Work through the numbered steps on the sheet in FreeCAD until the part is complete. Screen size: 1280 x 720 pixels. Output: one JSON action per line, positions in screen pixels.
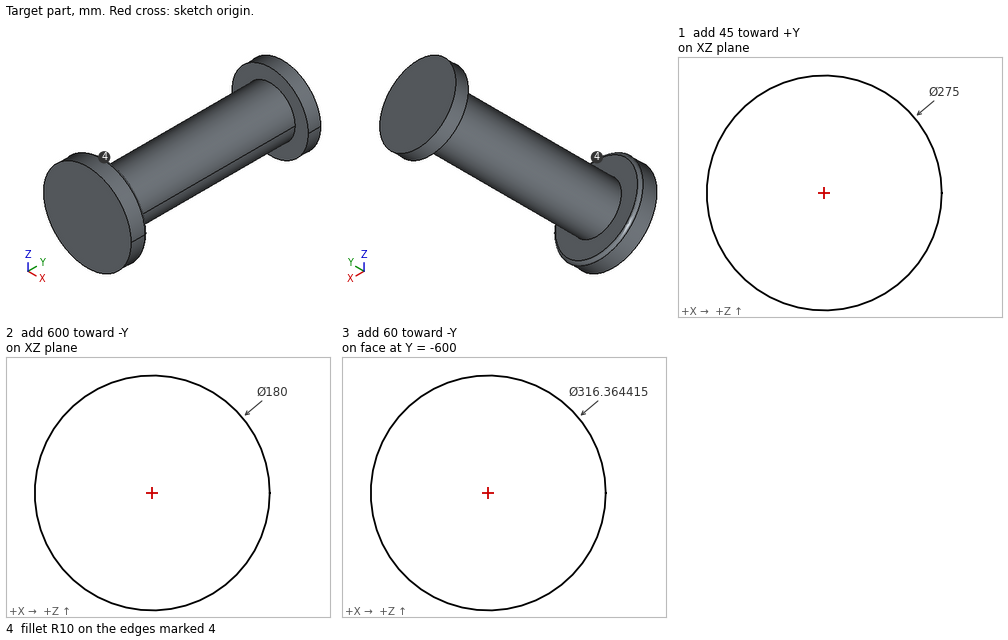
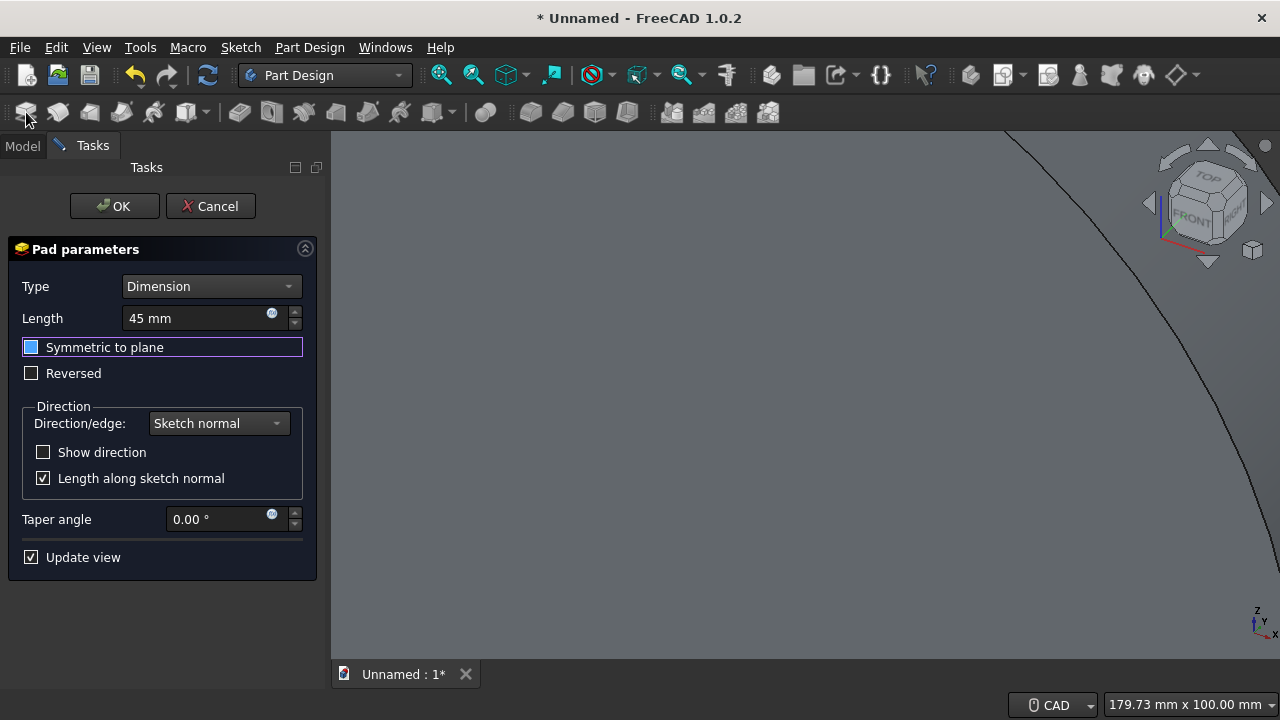
{"action": "left_click", "coordinate": [30, 373]}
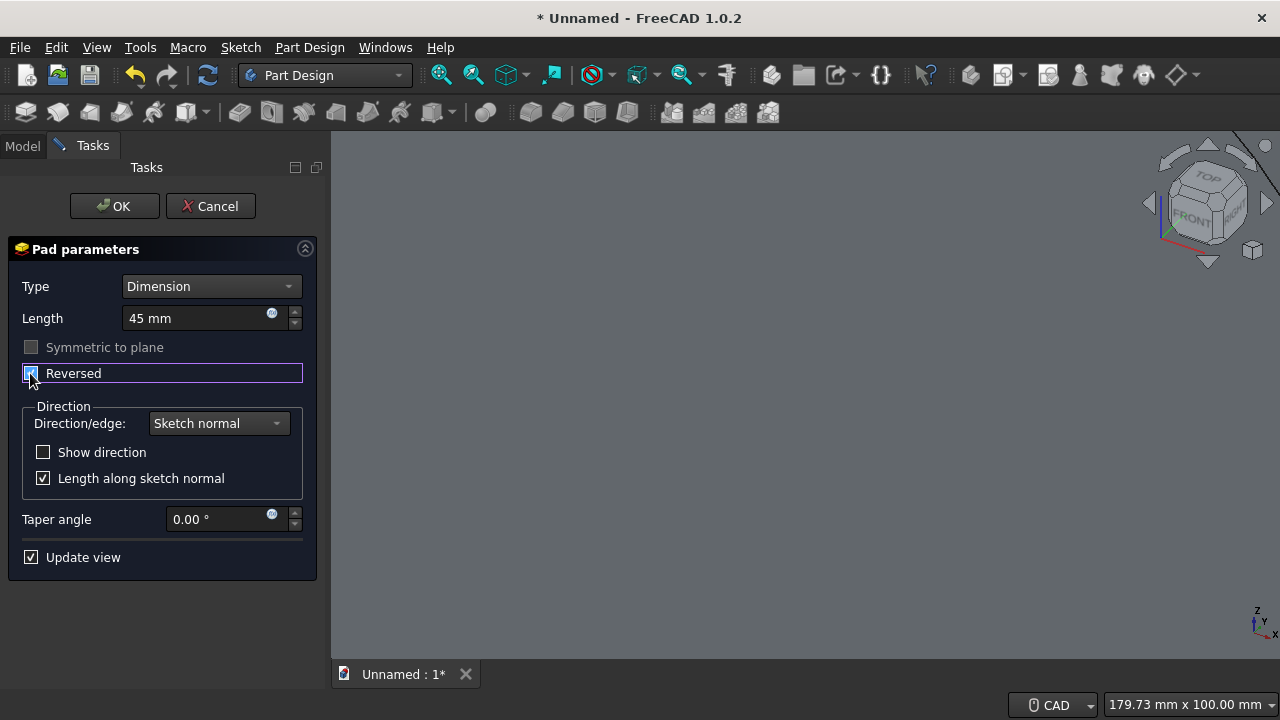
{"action": "left_click", "coordinate": [115, 206]}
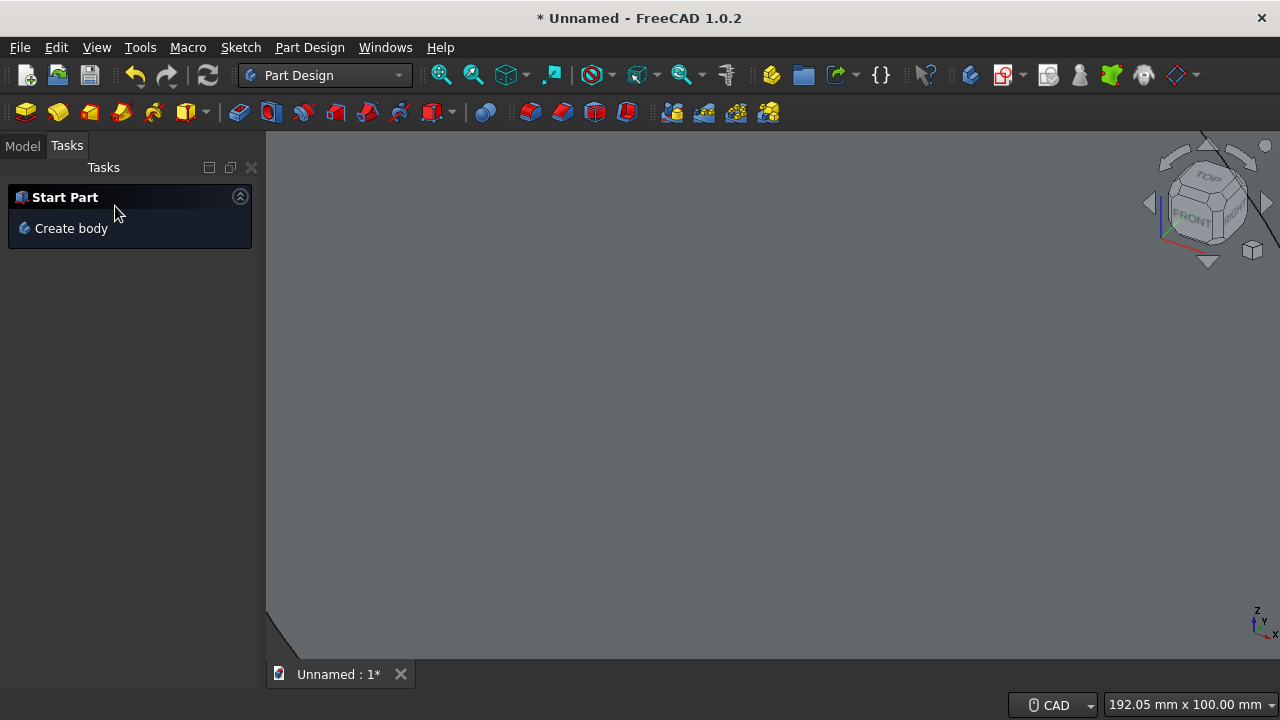
{"action": "key", "text": "v f"}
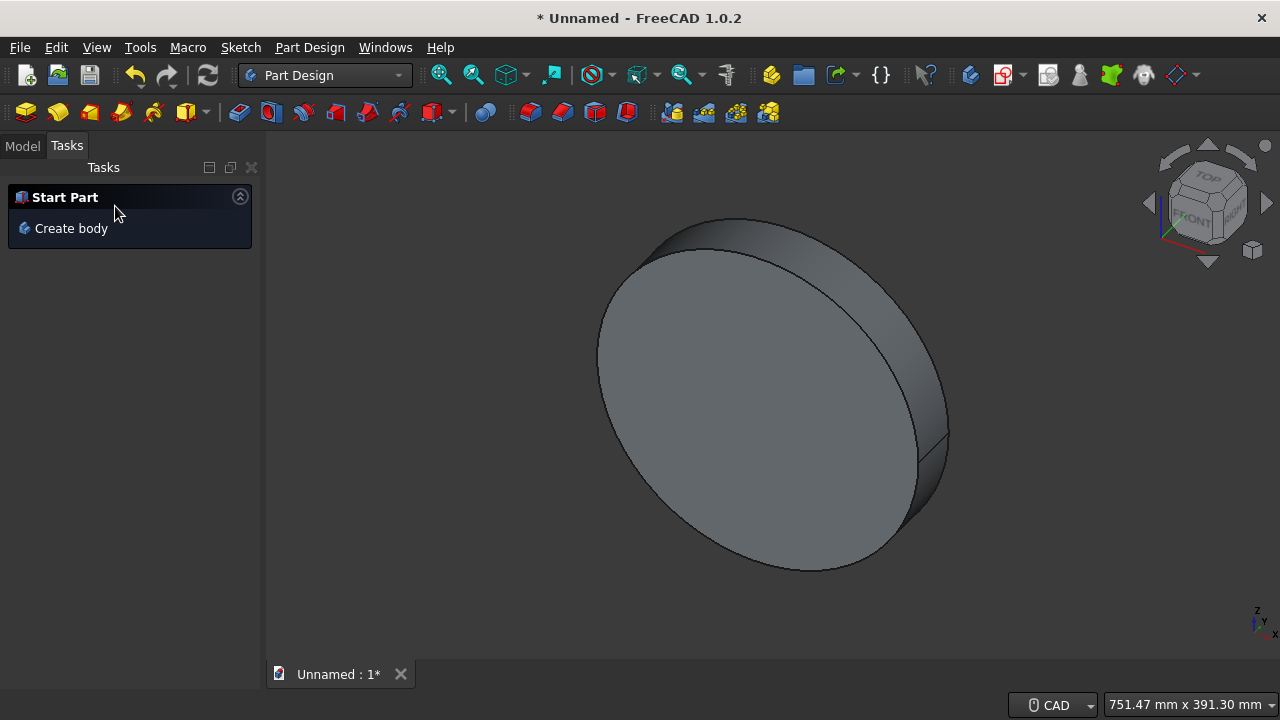
{"action": "left_click", "coordinate": [1004, 76]}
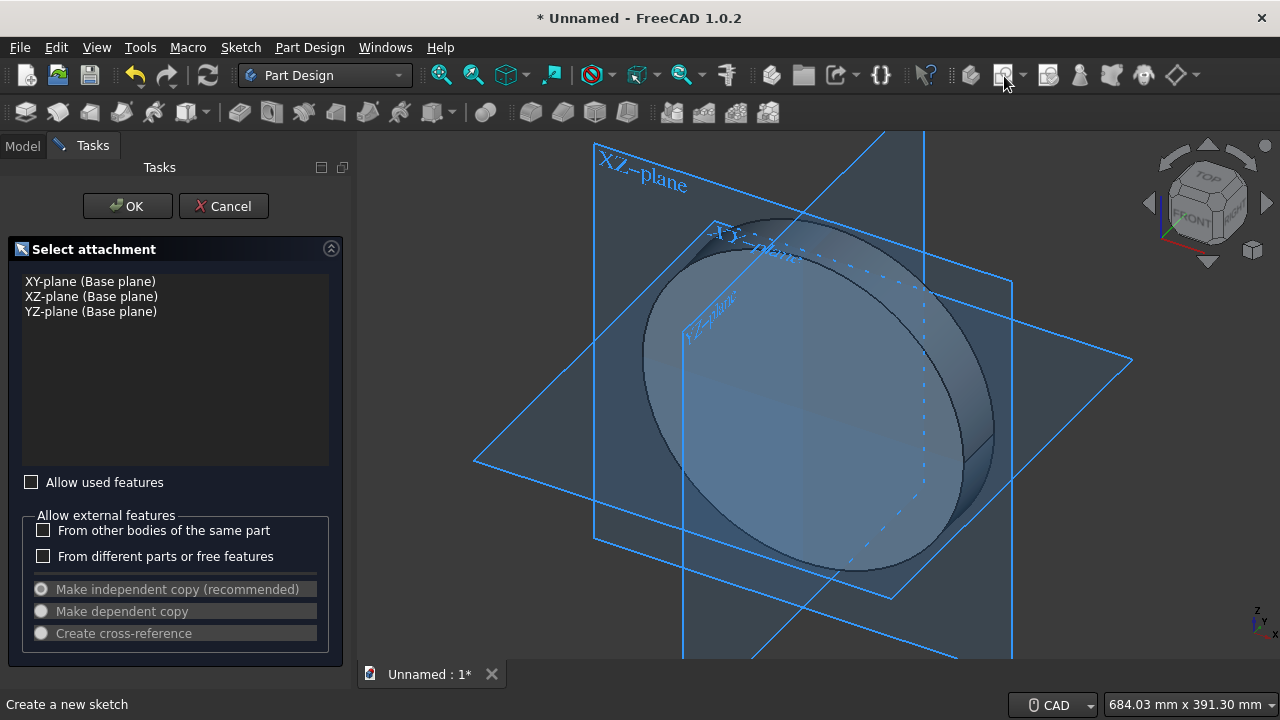
{"action": "left_click", "coordinate": [82, 296]}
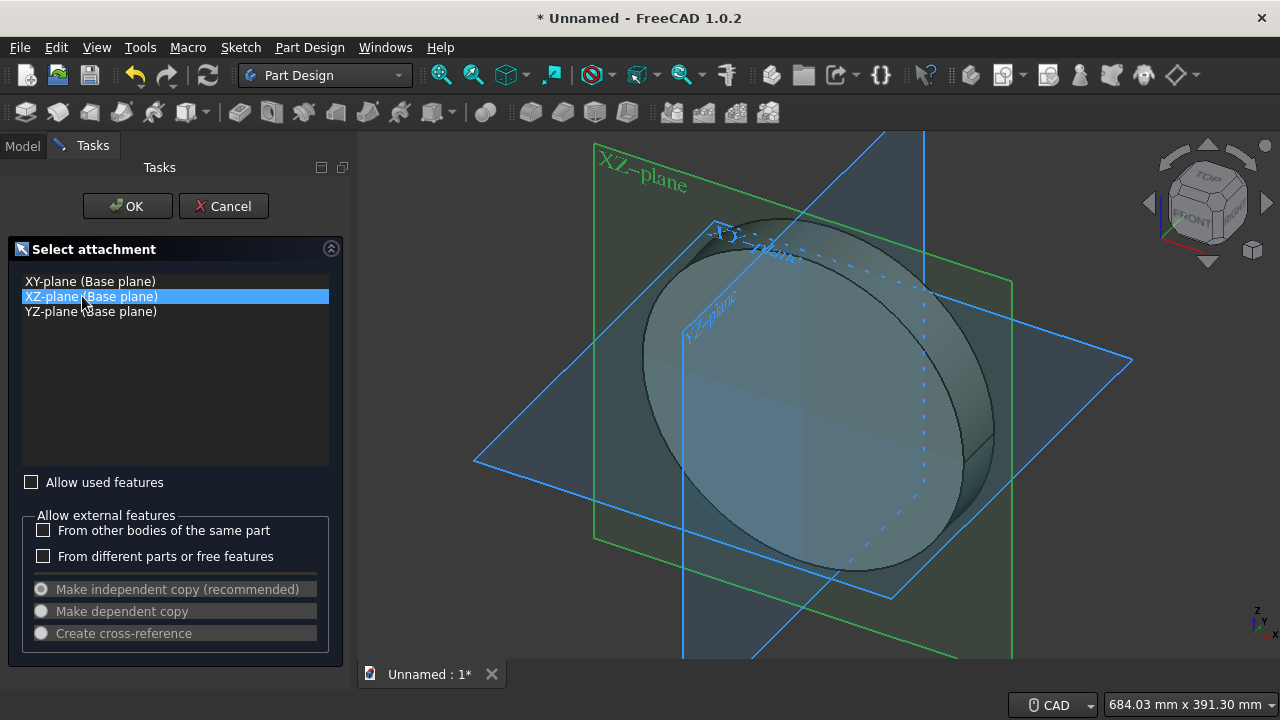
{"action": "left_click", "coordinate": [128, 206]}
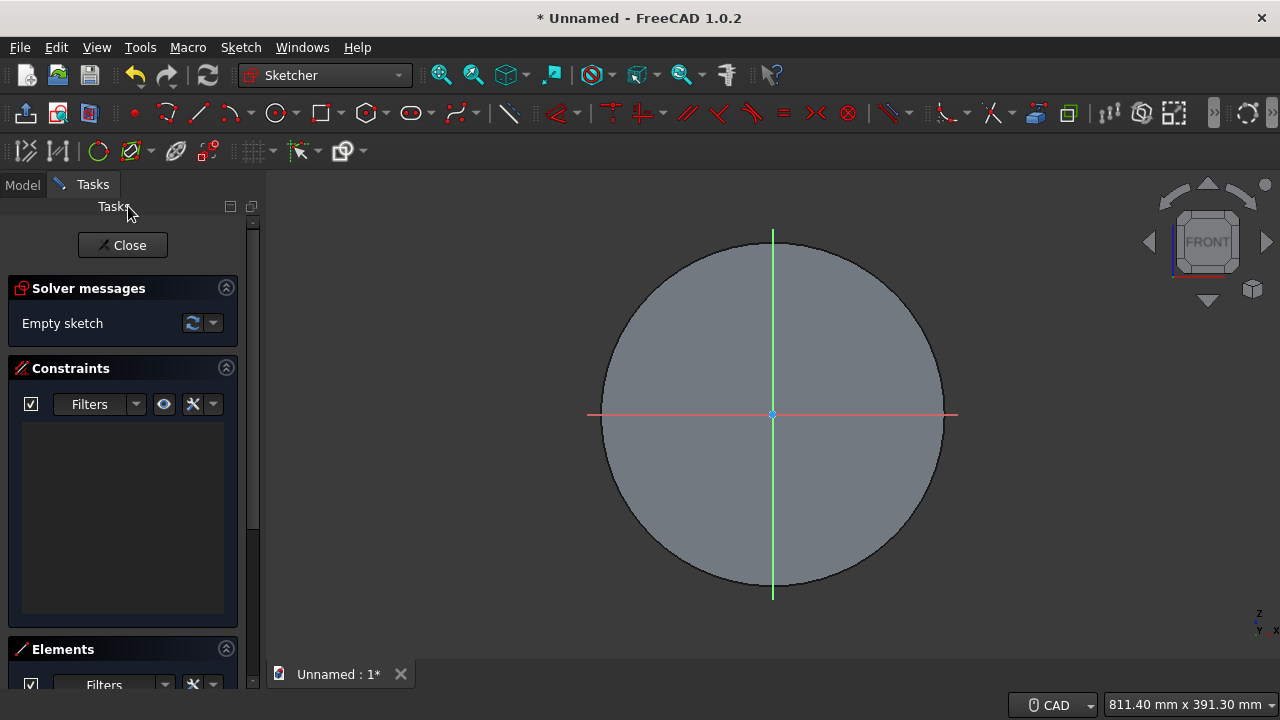
{"action": "scroll", "coordinate": [912, 414], "scroll_direction": "up", "scroll_amount": 2}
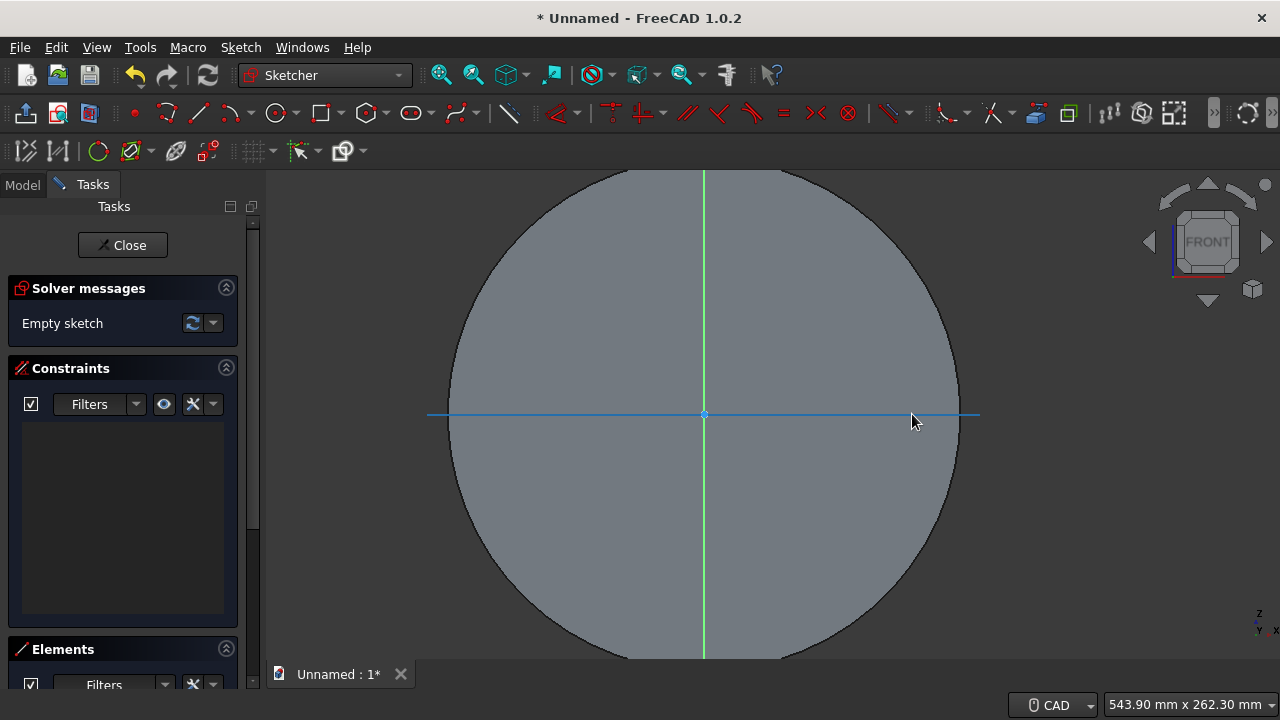
{"action": "key", "text": "g c"}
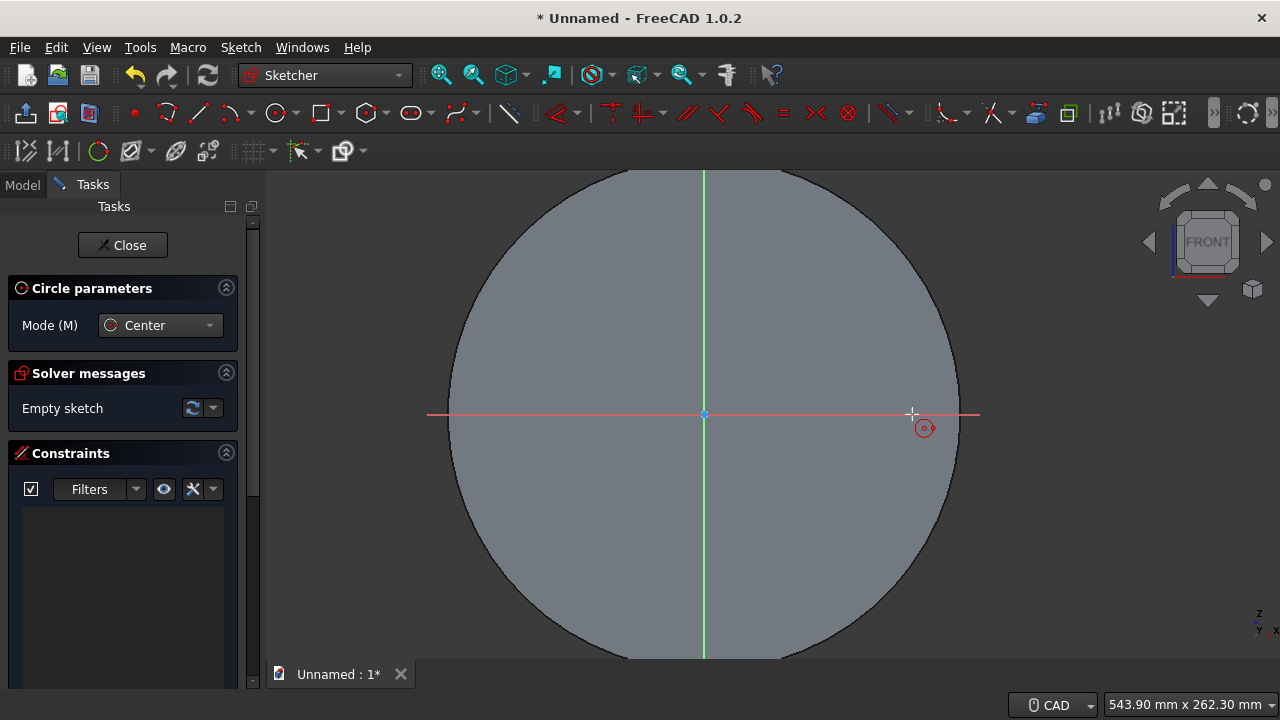
{"action": "left_click", "coordinate": [704, 414]}
{"action": "mouse_move", "coordinate": [823, 296]}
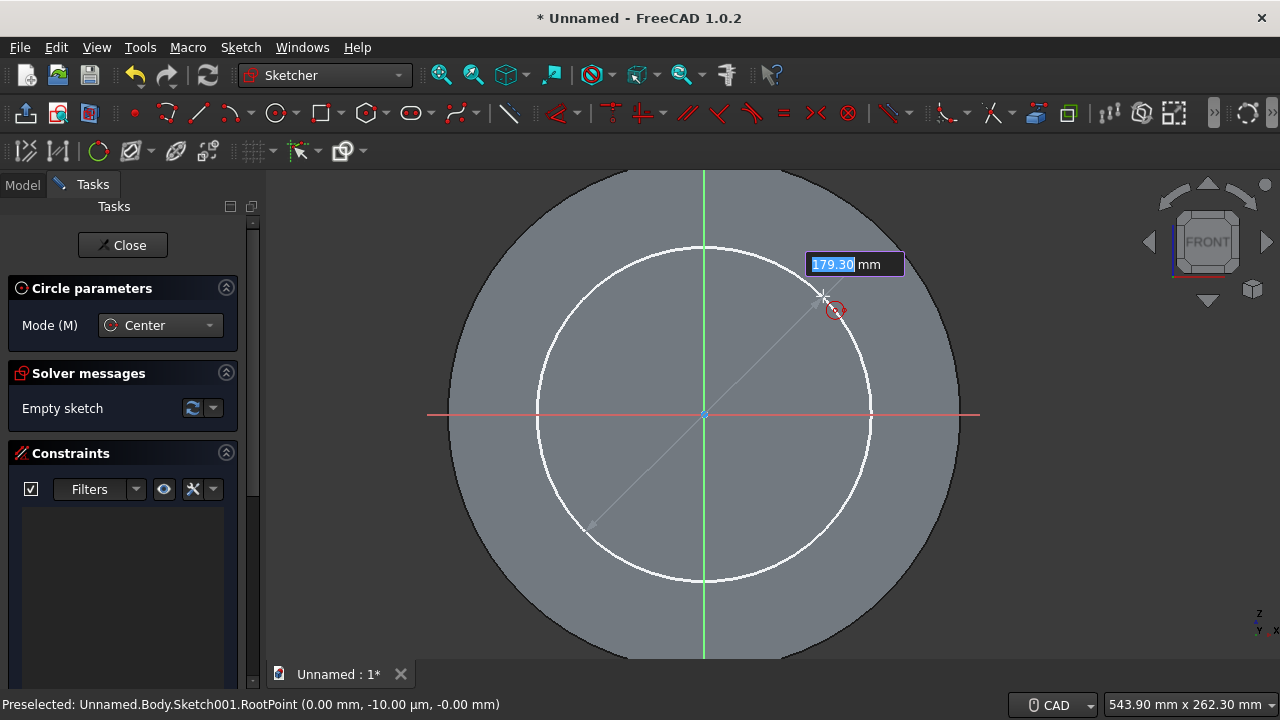
{"action": "type", "text": "180"}
{"action": "key", "text": "Return"}
{"action": "key", "text": "Escape"}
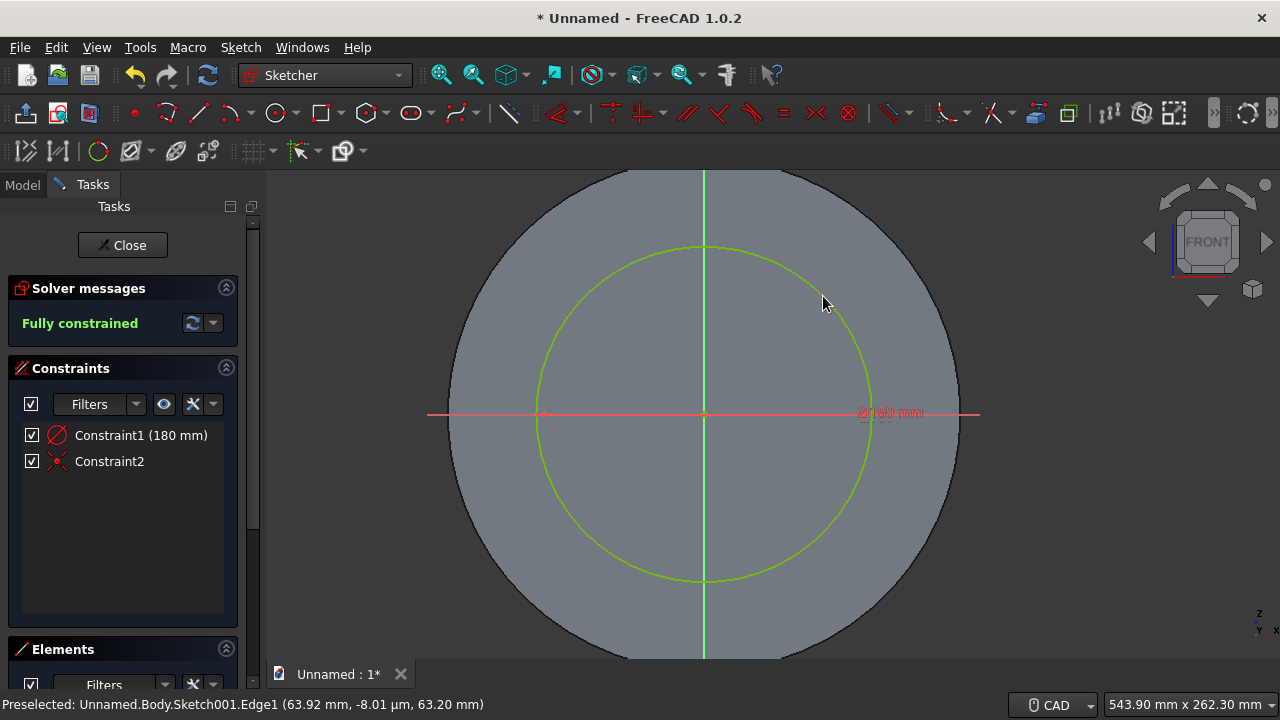
{"action": "left_click", "coordinate": [123, 245]}